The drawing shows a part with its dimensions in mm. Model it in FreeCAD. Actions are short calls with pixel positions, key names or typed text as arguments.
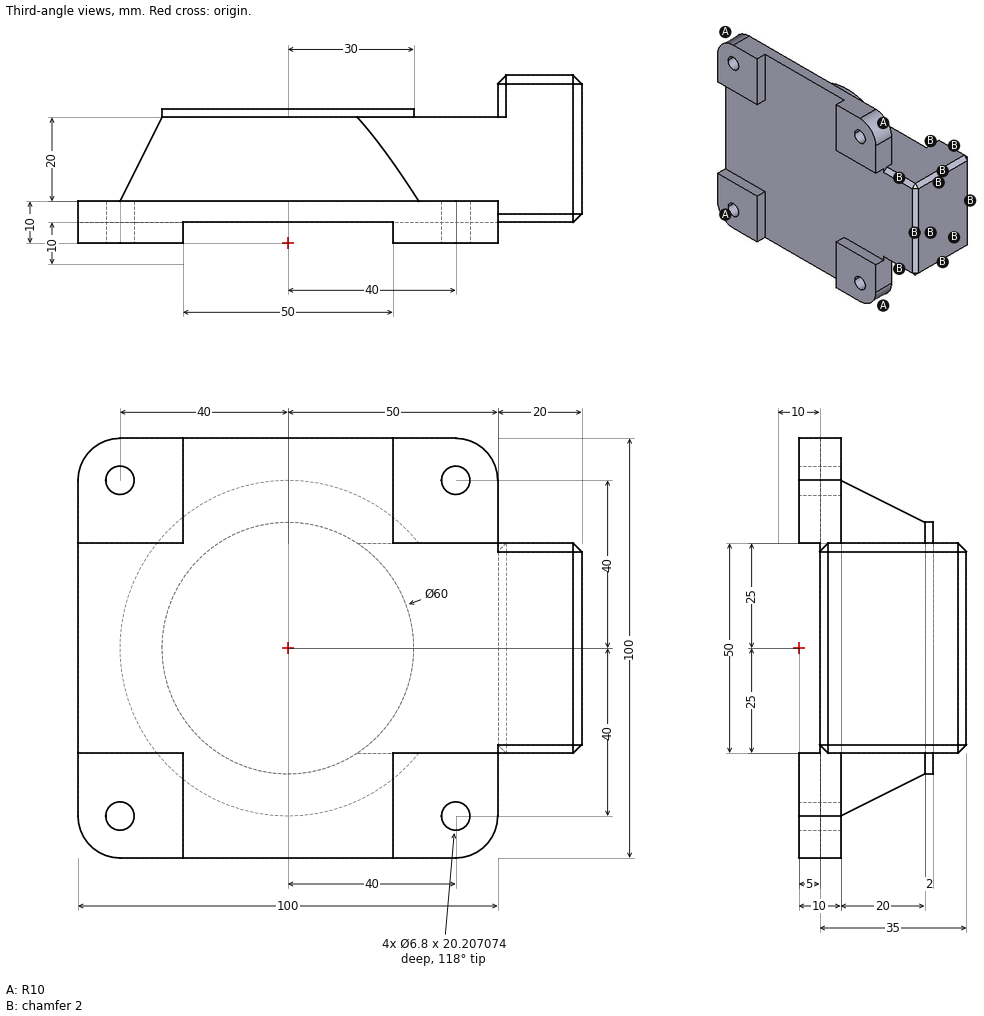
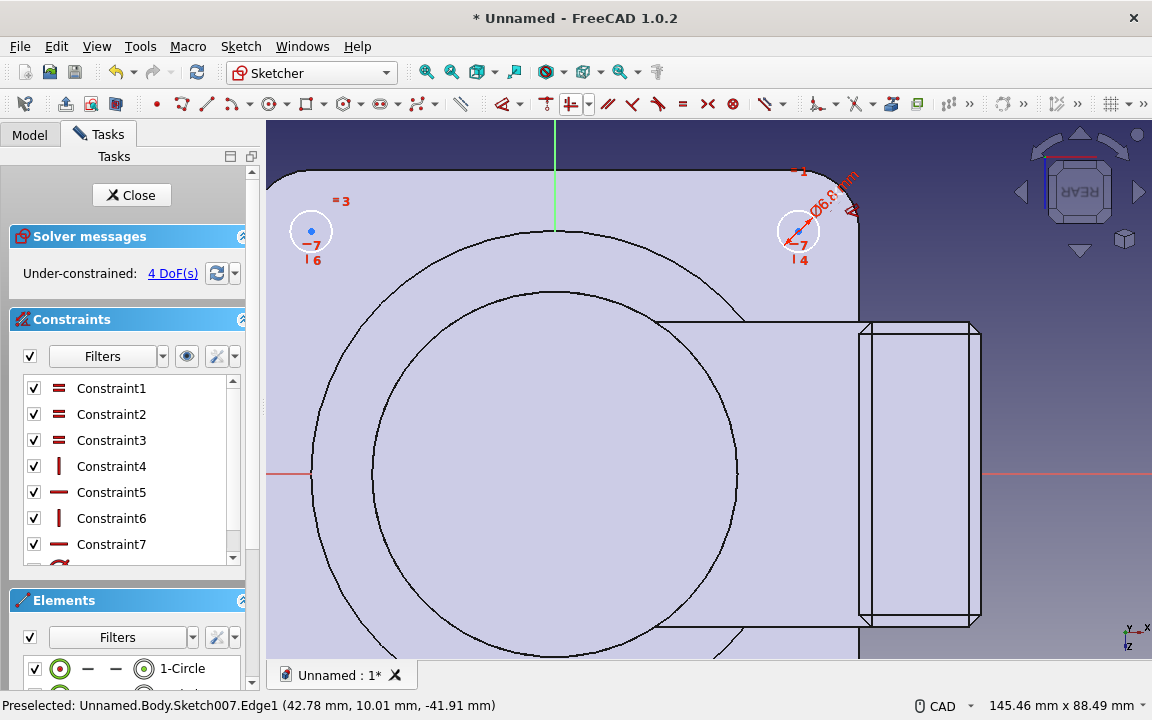
click(799, 231)
click(677, 197)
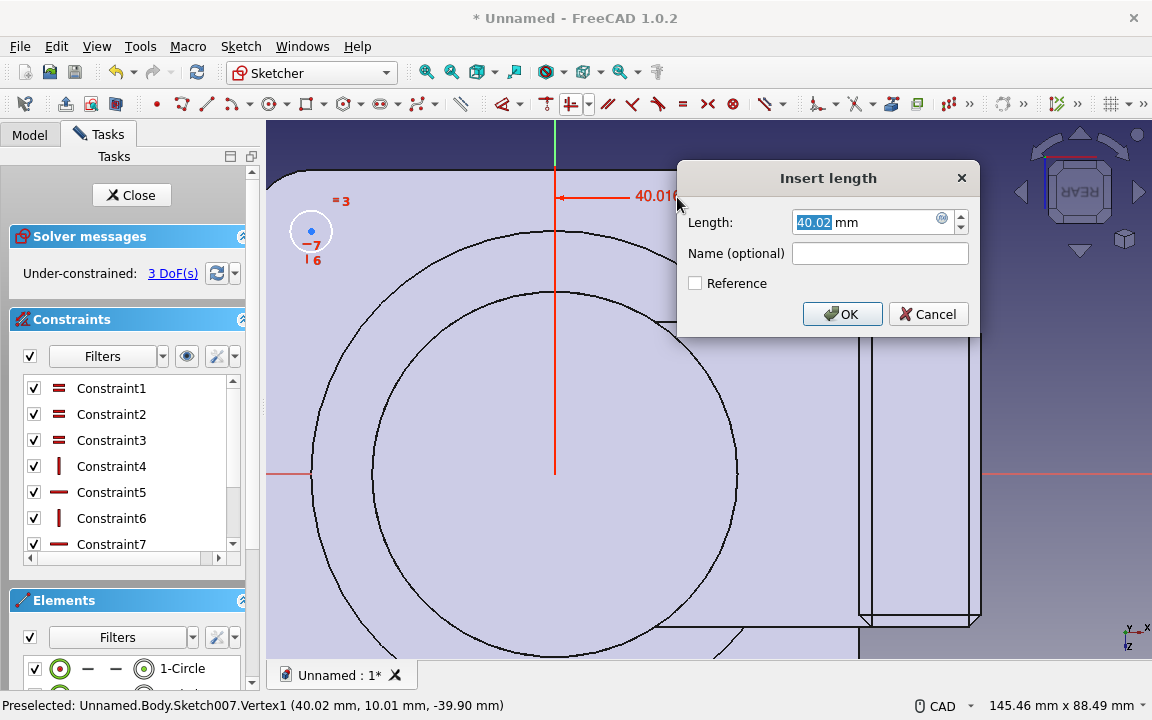
text(40)
key(Return)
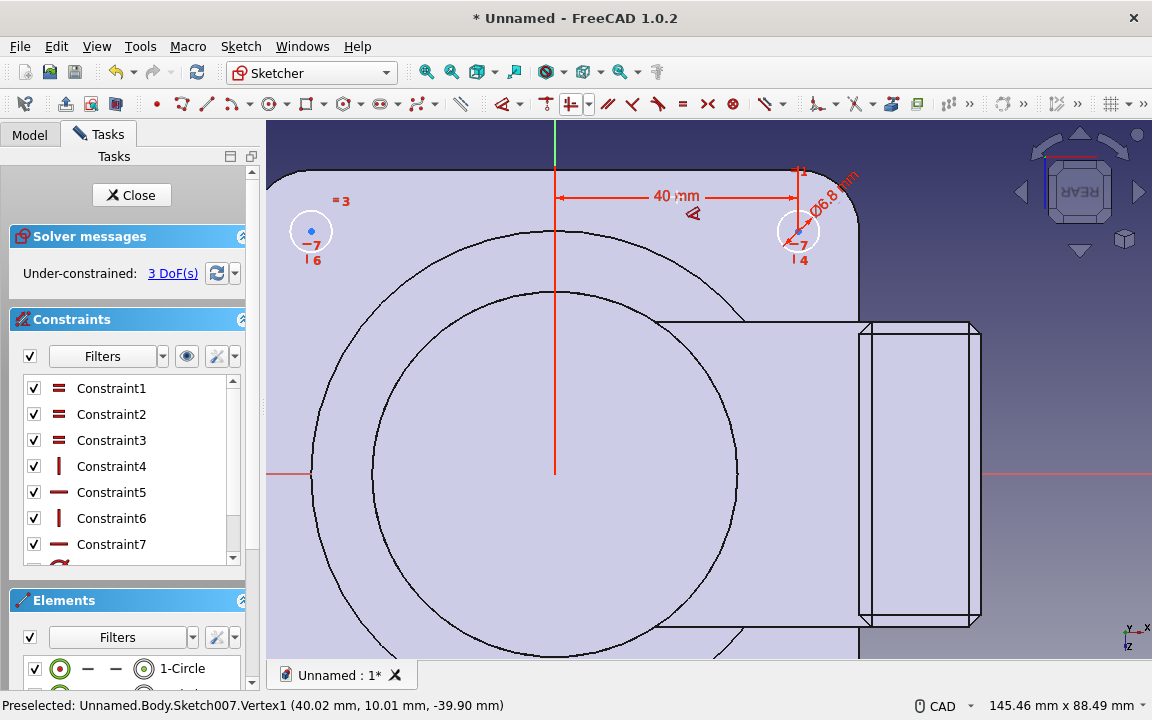
click(798, 231)
click(832, 353)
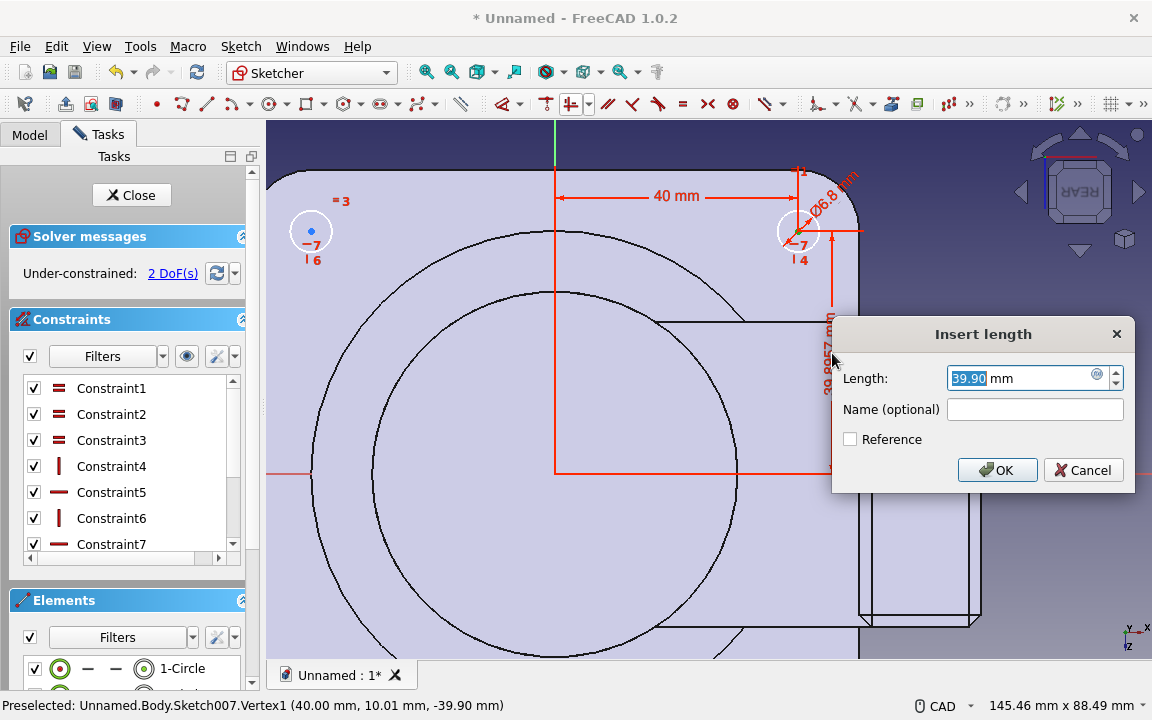
text(40)
key(Return)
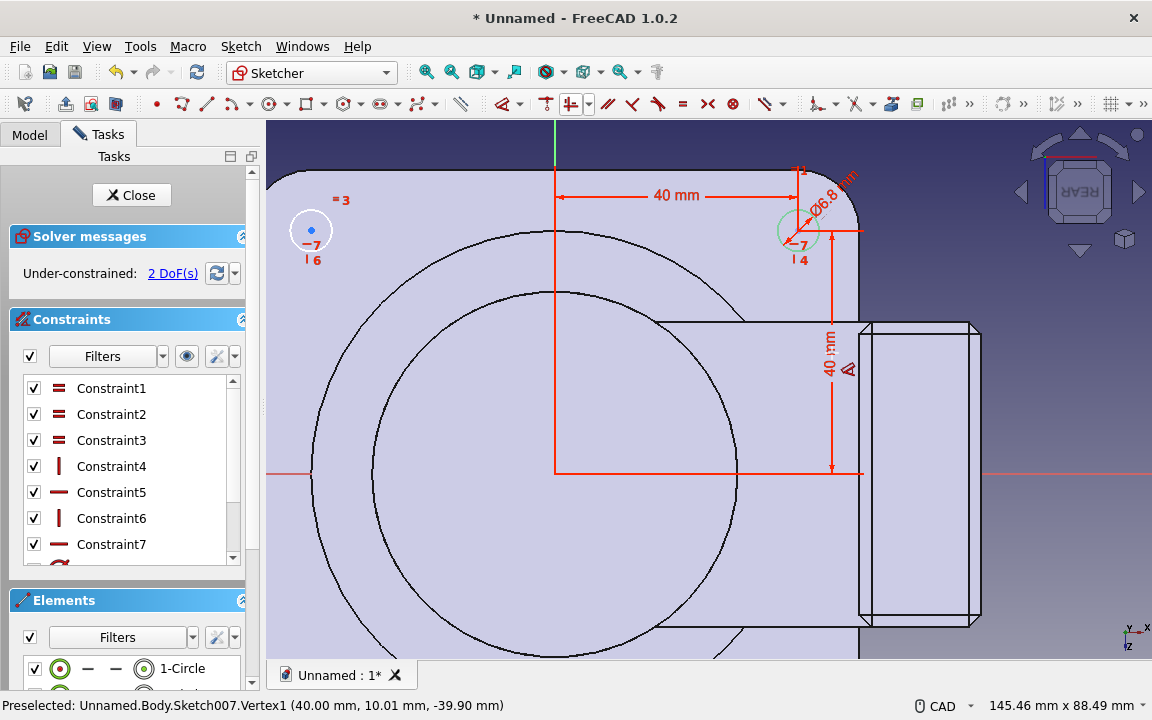
scroll(815, 217, down, 2)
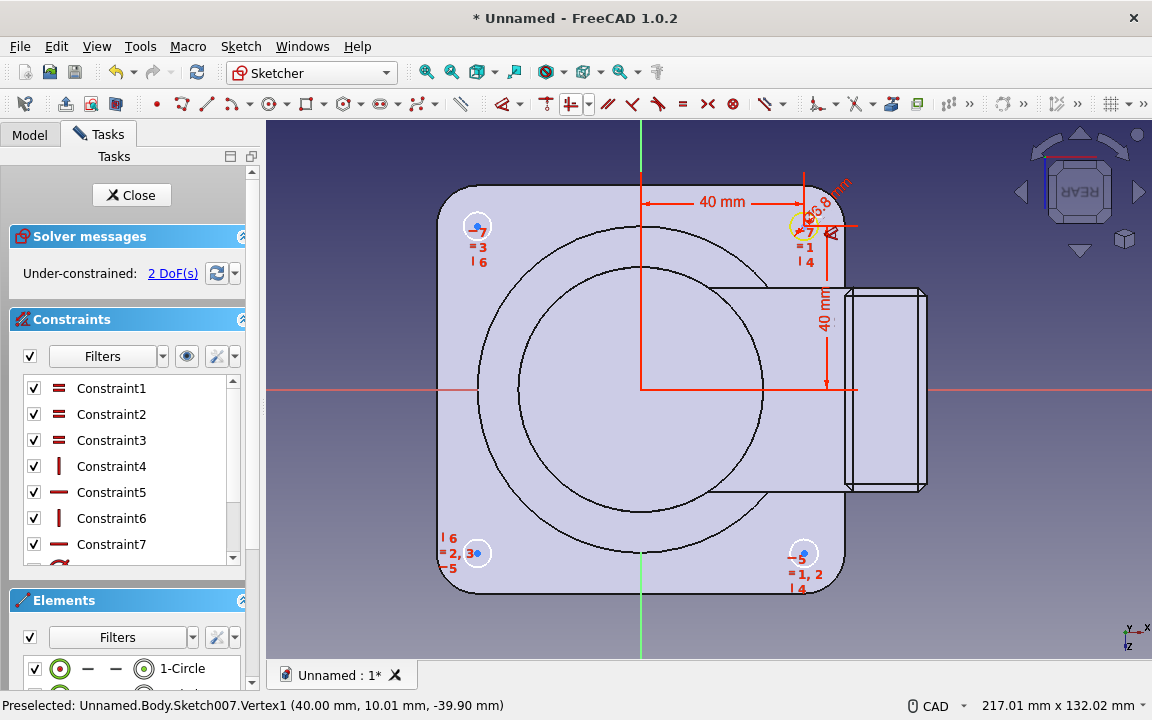
click(804, 553)
click(838, 471)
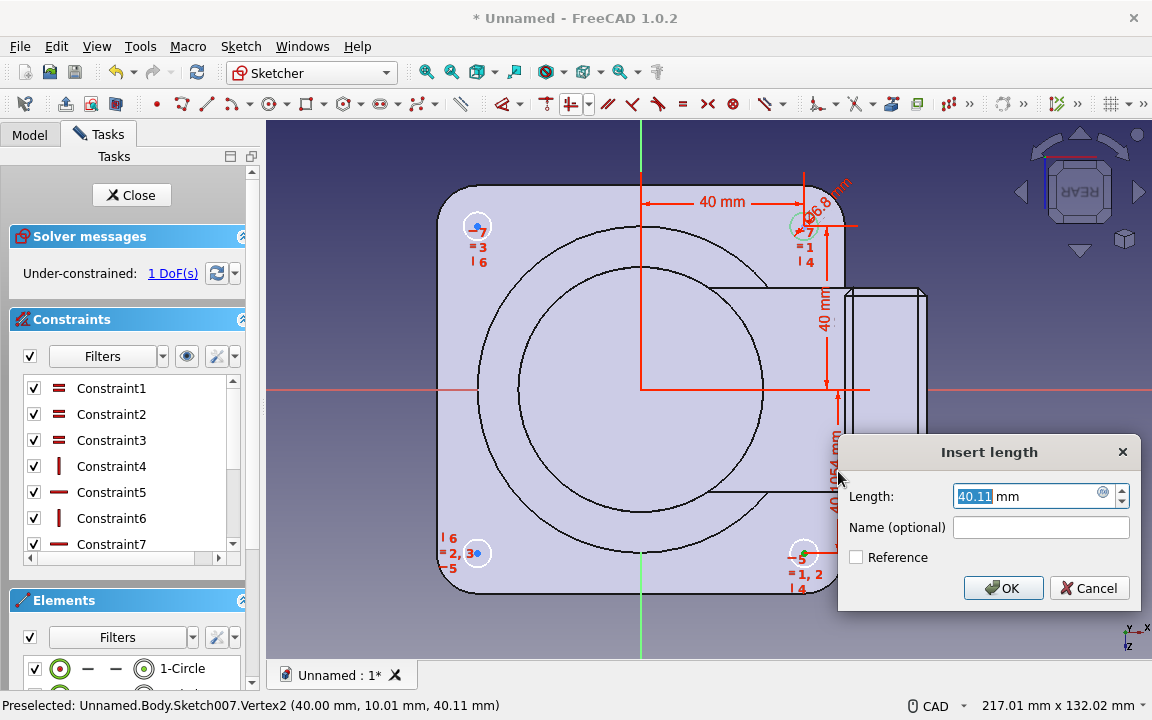
text(40)
key(Return)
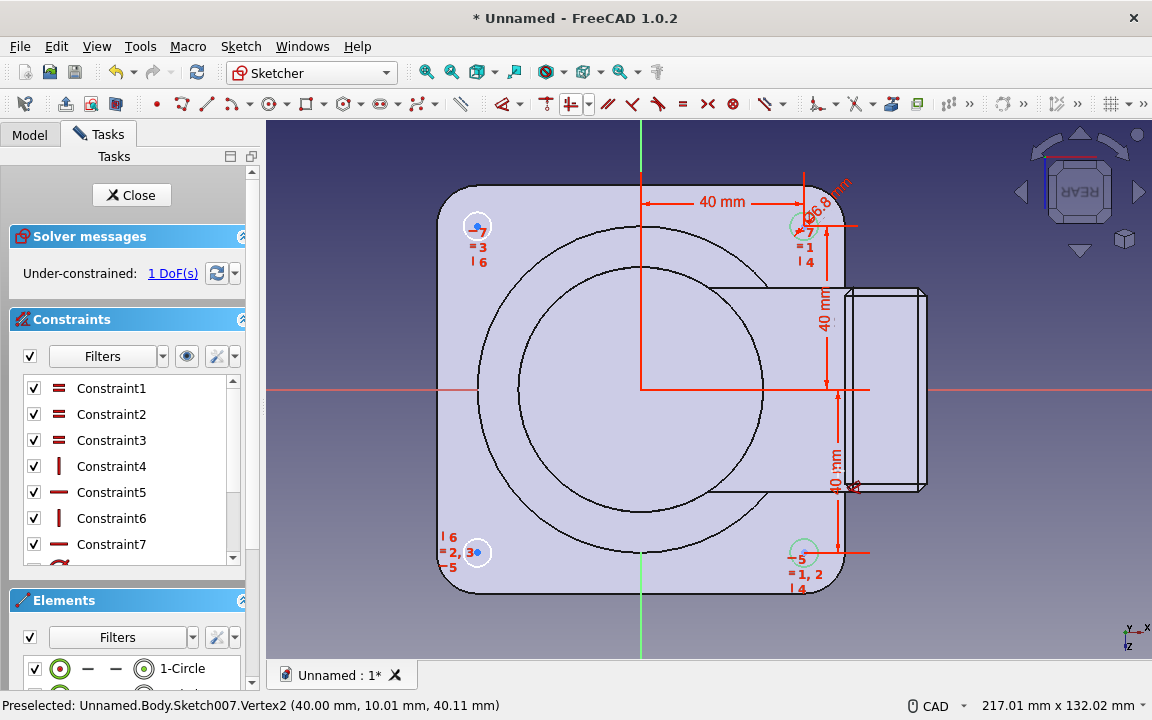
click(477, 553)
click(559, 587)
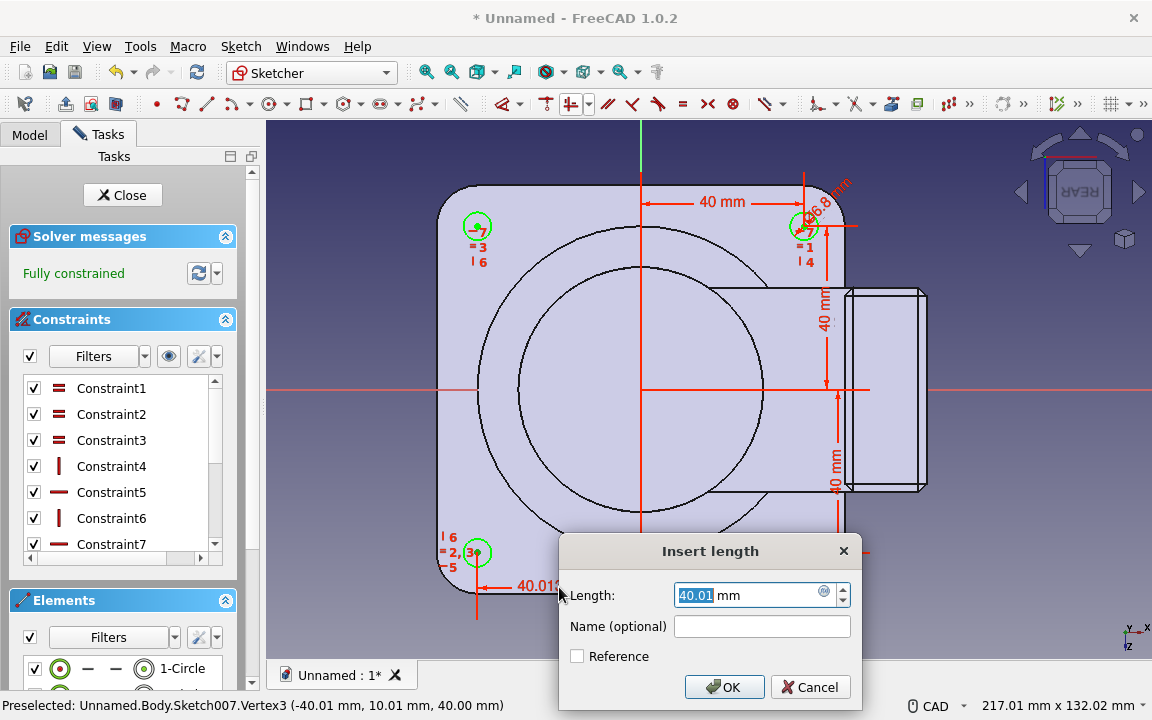
text(40)
key(Return)
key(Escape)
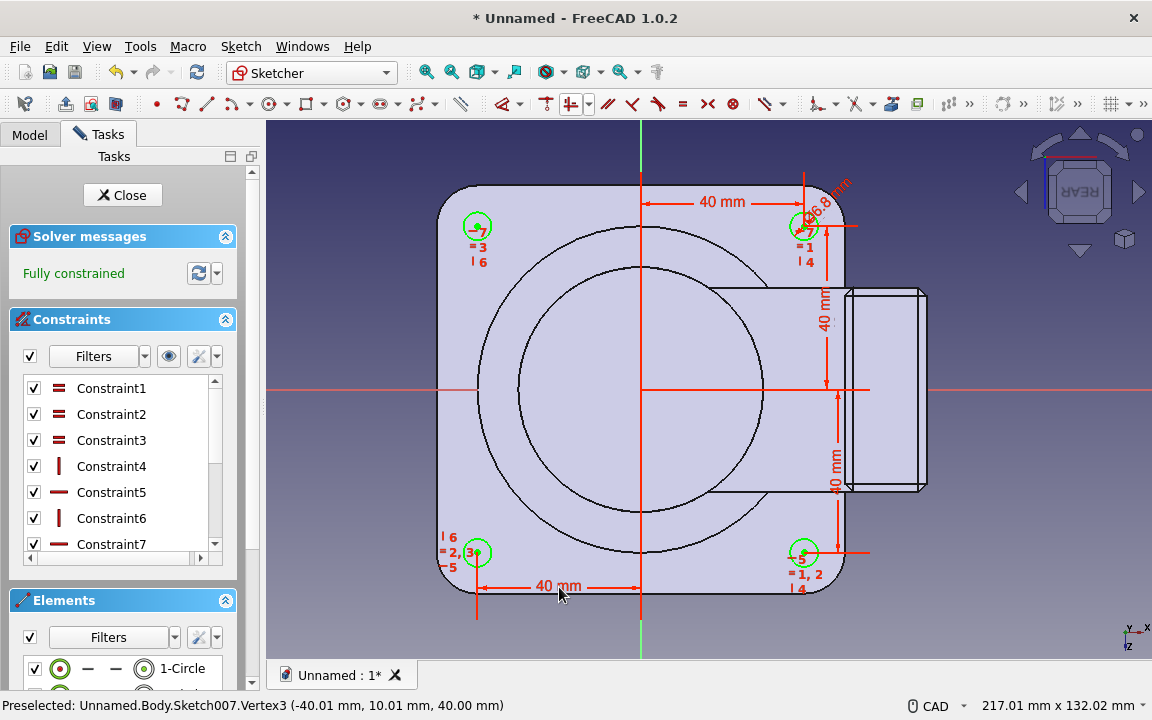
click(123, 195)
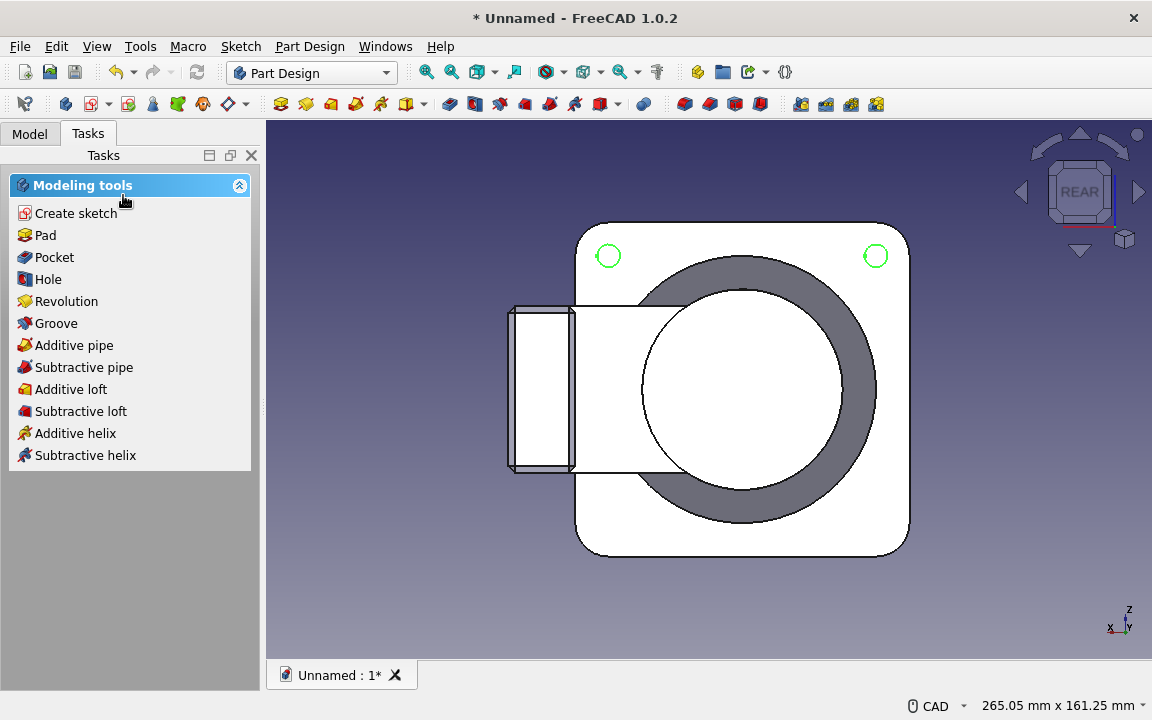
click(475, 104)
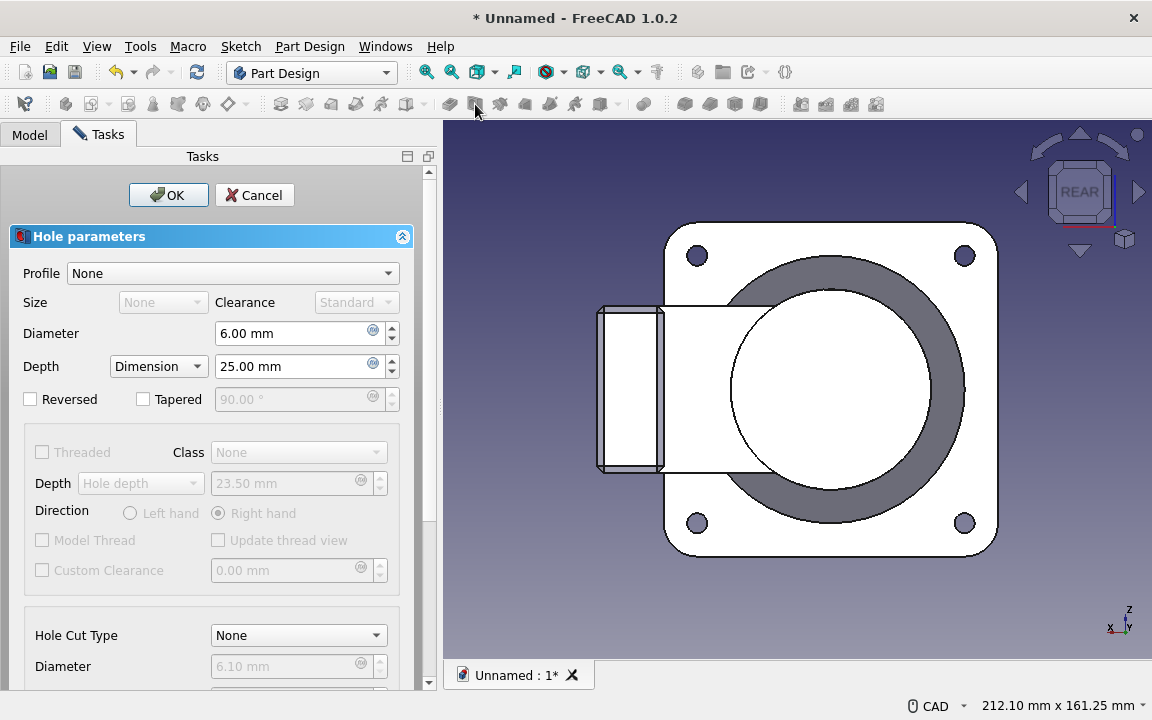
triple_click(300, 334)